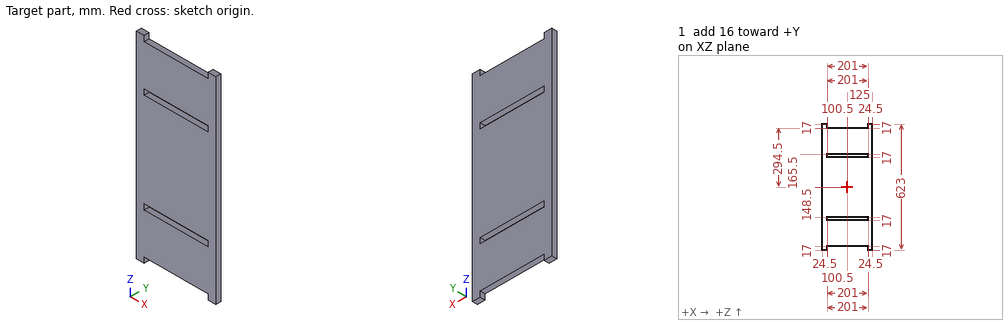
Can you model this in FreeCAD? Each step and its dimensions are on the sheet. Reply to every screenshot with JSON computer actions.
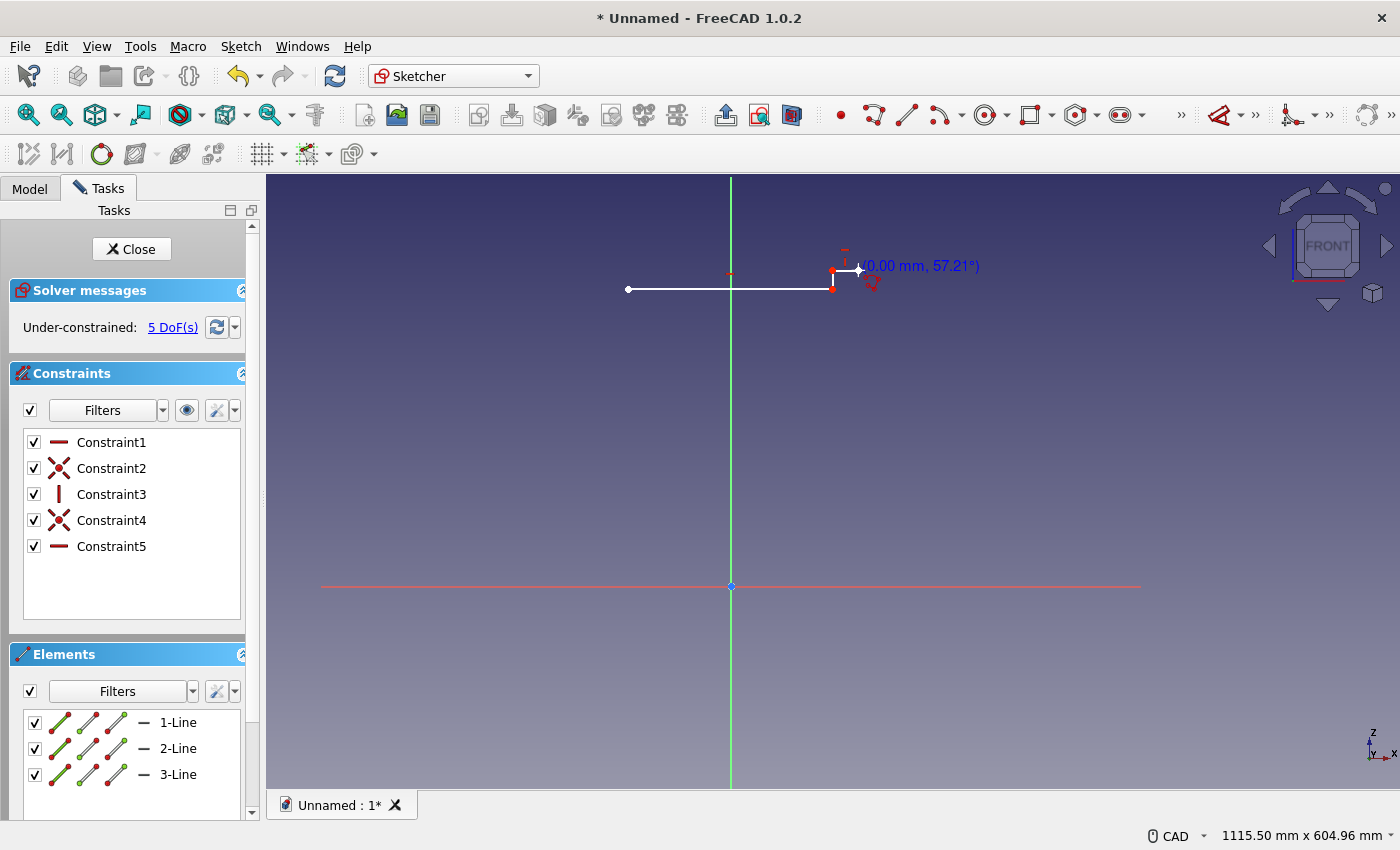
{"action": "scroll", "coordinate": [832, 267], "scroll_direction": "down", "scroll_amount": 2}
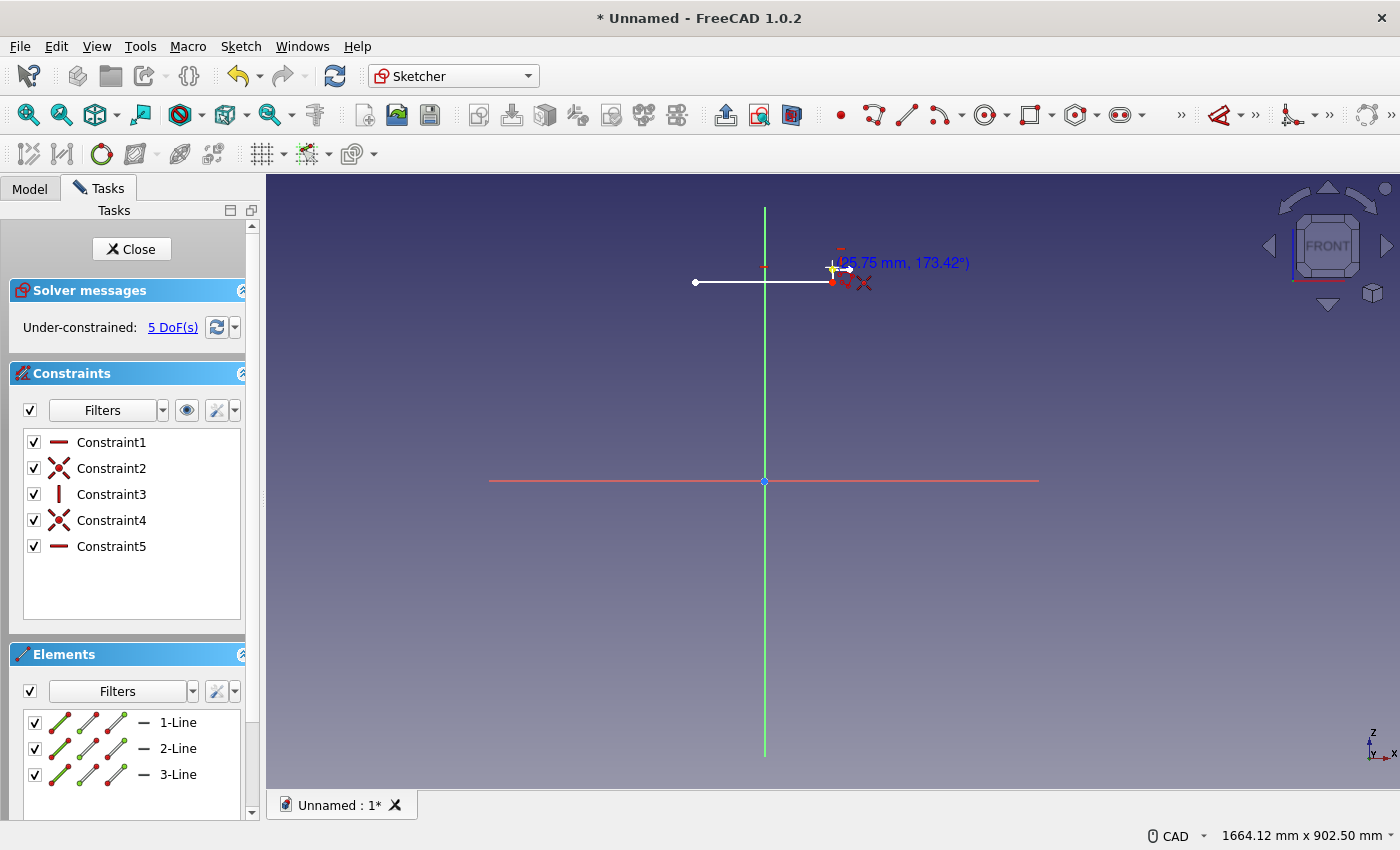
{"action": "left_click", "coordinate": [850, 694]}
{"action": "left_click", "coordinate": [833, 694]}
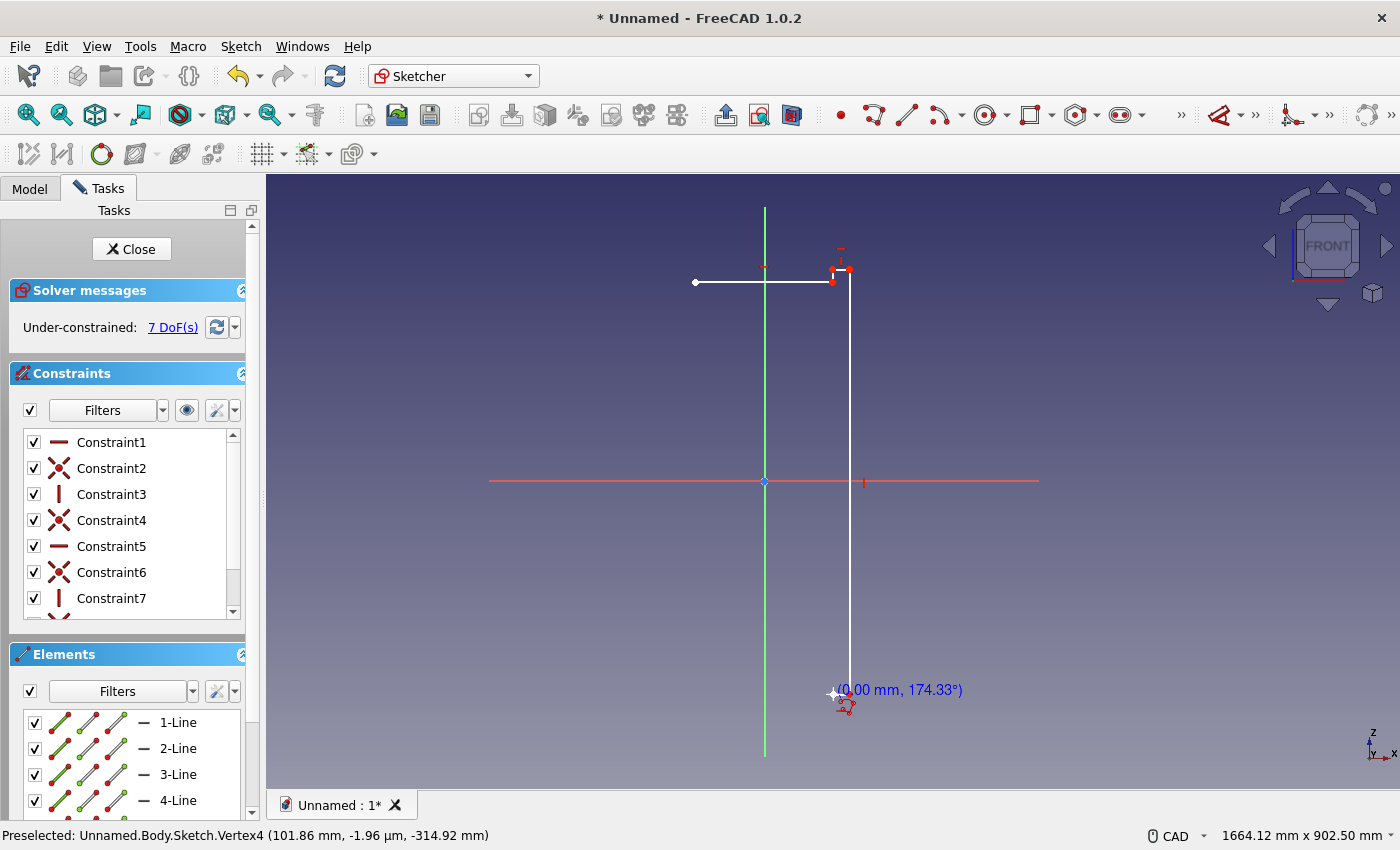
{"action": "scroll", "coordinate": [833, 682], "scroll_direction": "up", "scroll_amount": 2}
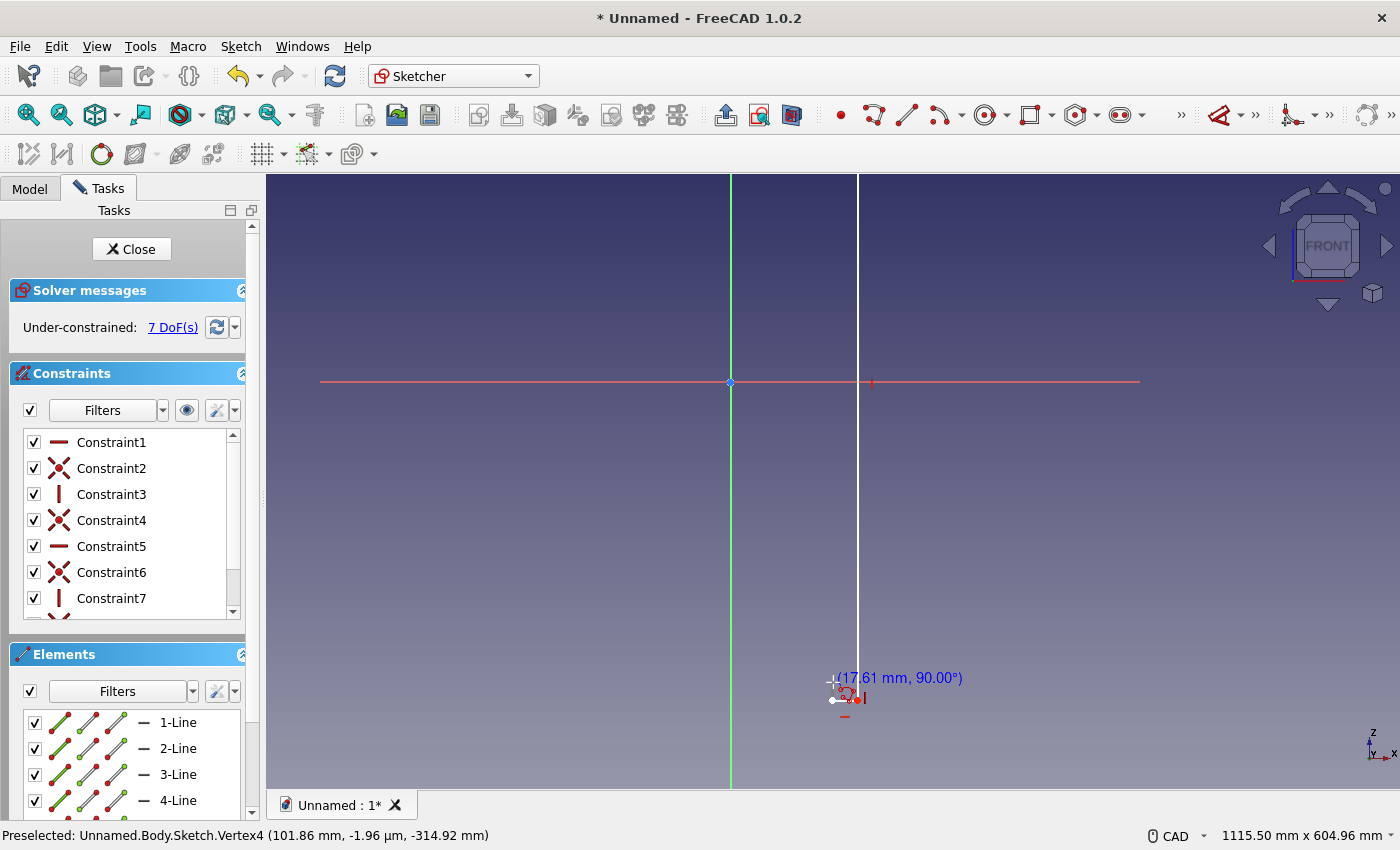
{"action": "left_click", "coordinate": [833, 682]}
{"action": "left_click", "coordinate": [629, 682]}
{"action": "left_click", "coordinate": [629, 699]}
{"action": "left_click", "coordinate": [604, 699]}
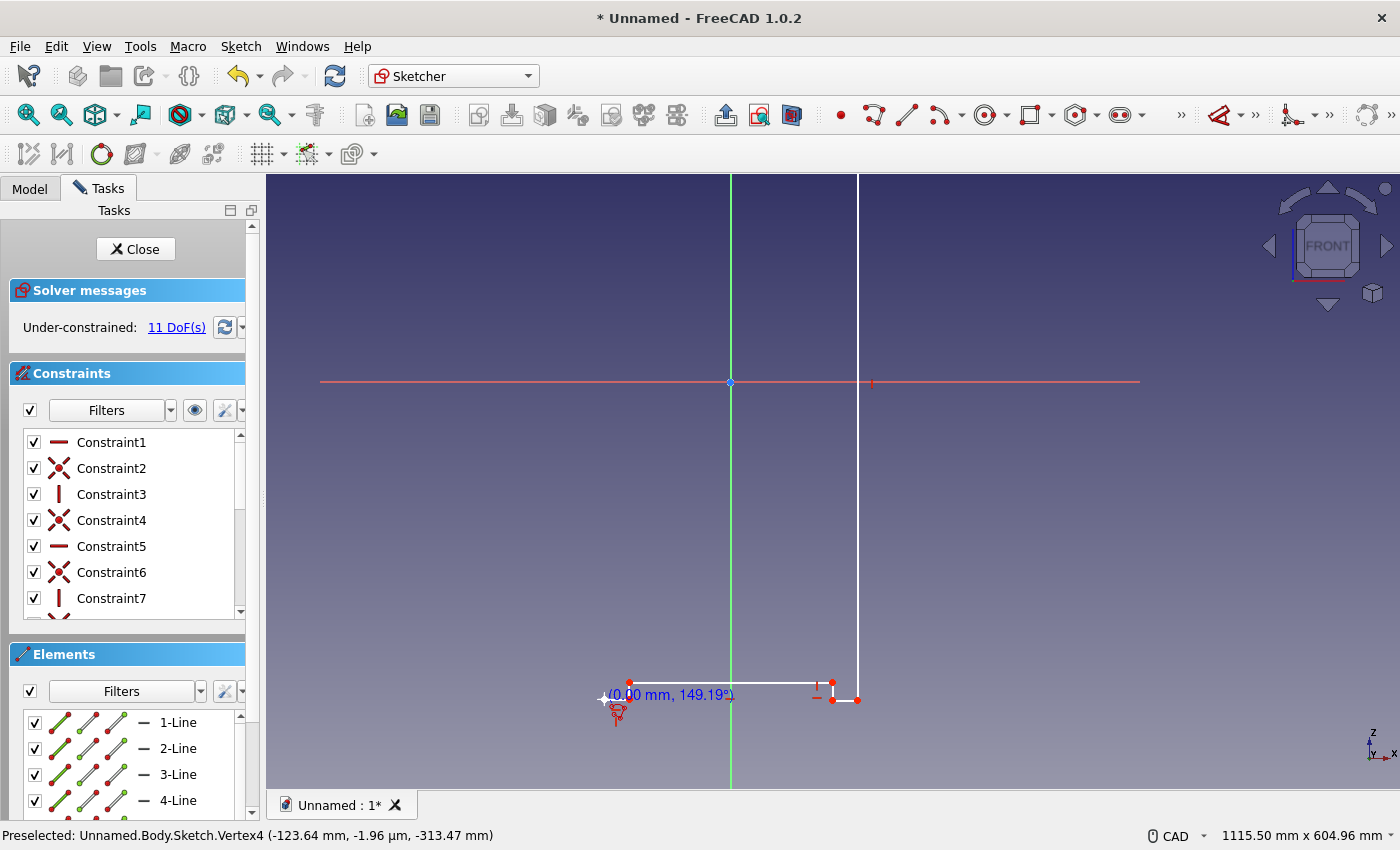
{"action": "scroll", "coordinate": [833, 683], "scroll_direction": "down", "scroll_amount": 2}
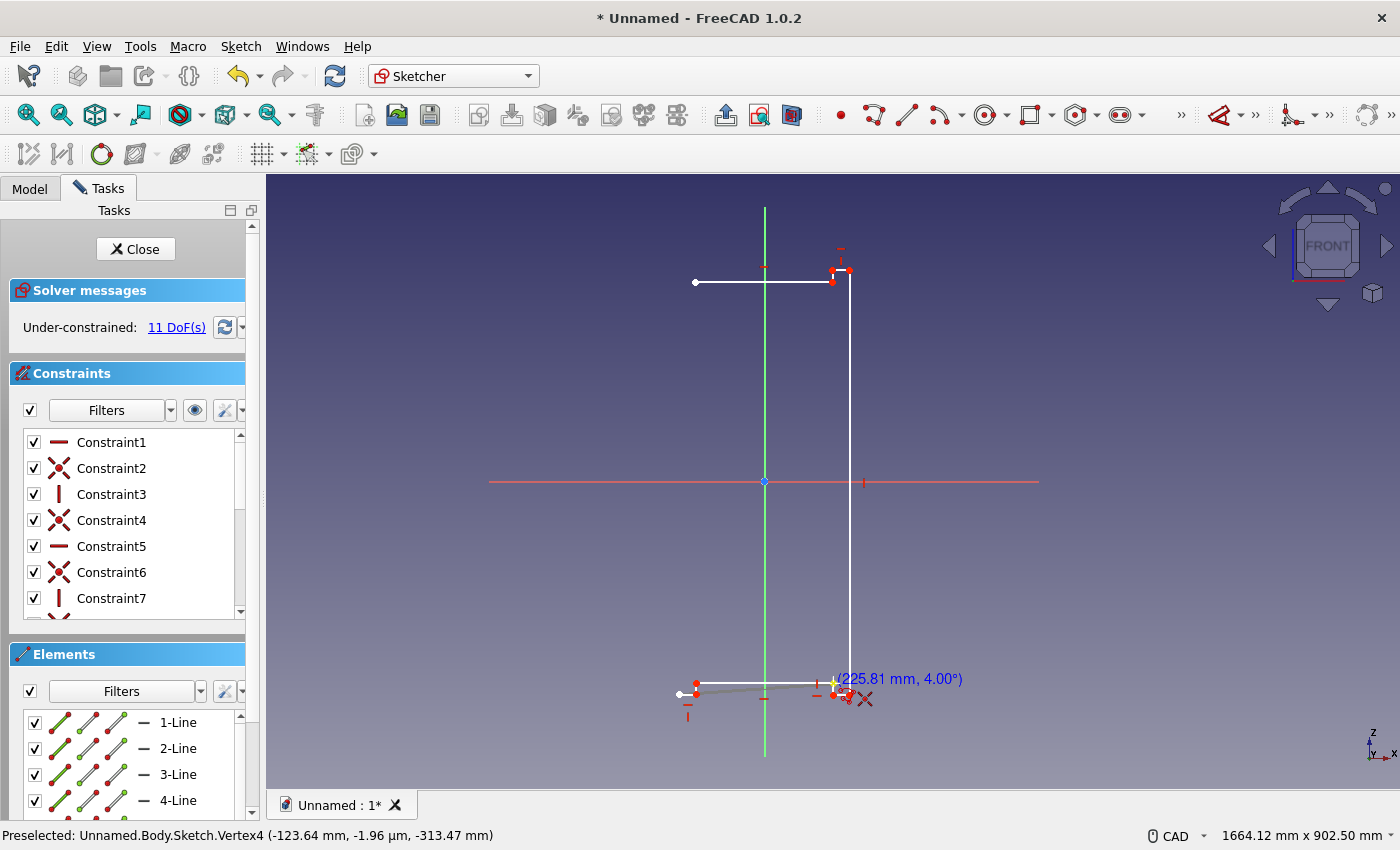
{"action": "left_click", "coordinate": [680, 269]}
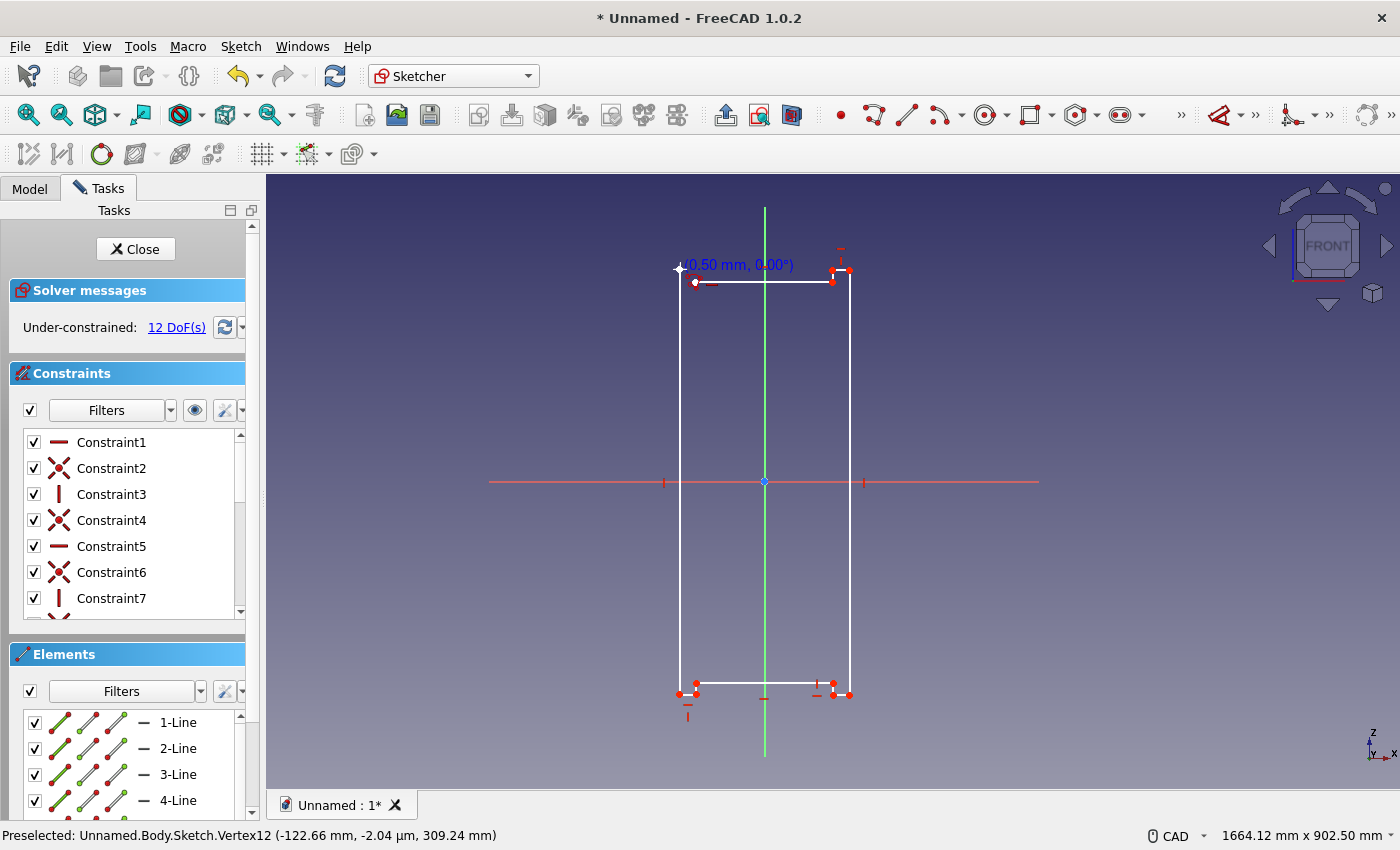
{"action": "scroll", "coordinate": [696, 269], "scroll_direction": "up", "scroll_amount": 2}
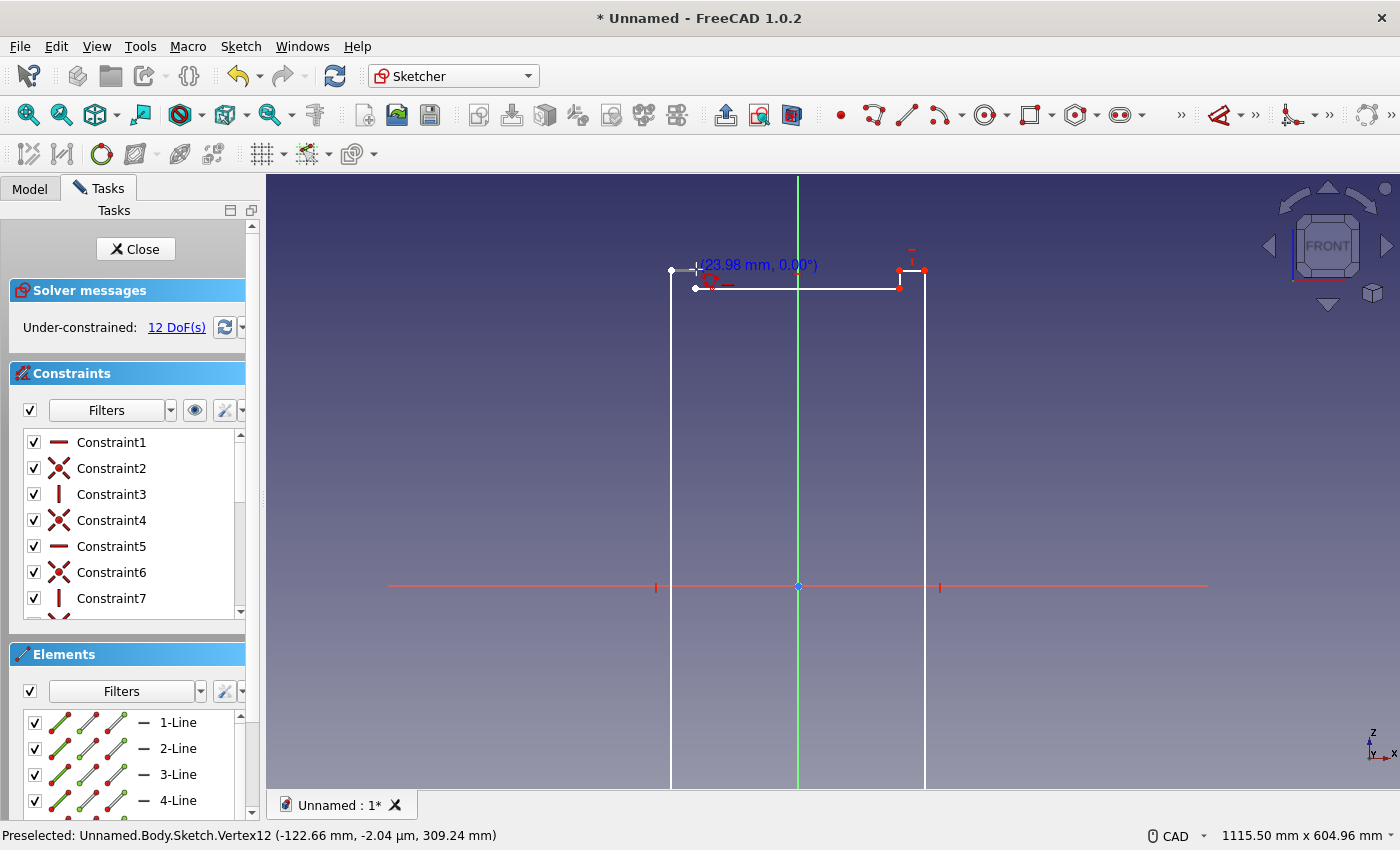
{"action": "left_click", "coordinate": [696, 269]}
{"action": "left_click", "coordinate": [695, 289]}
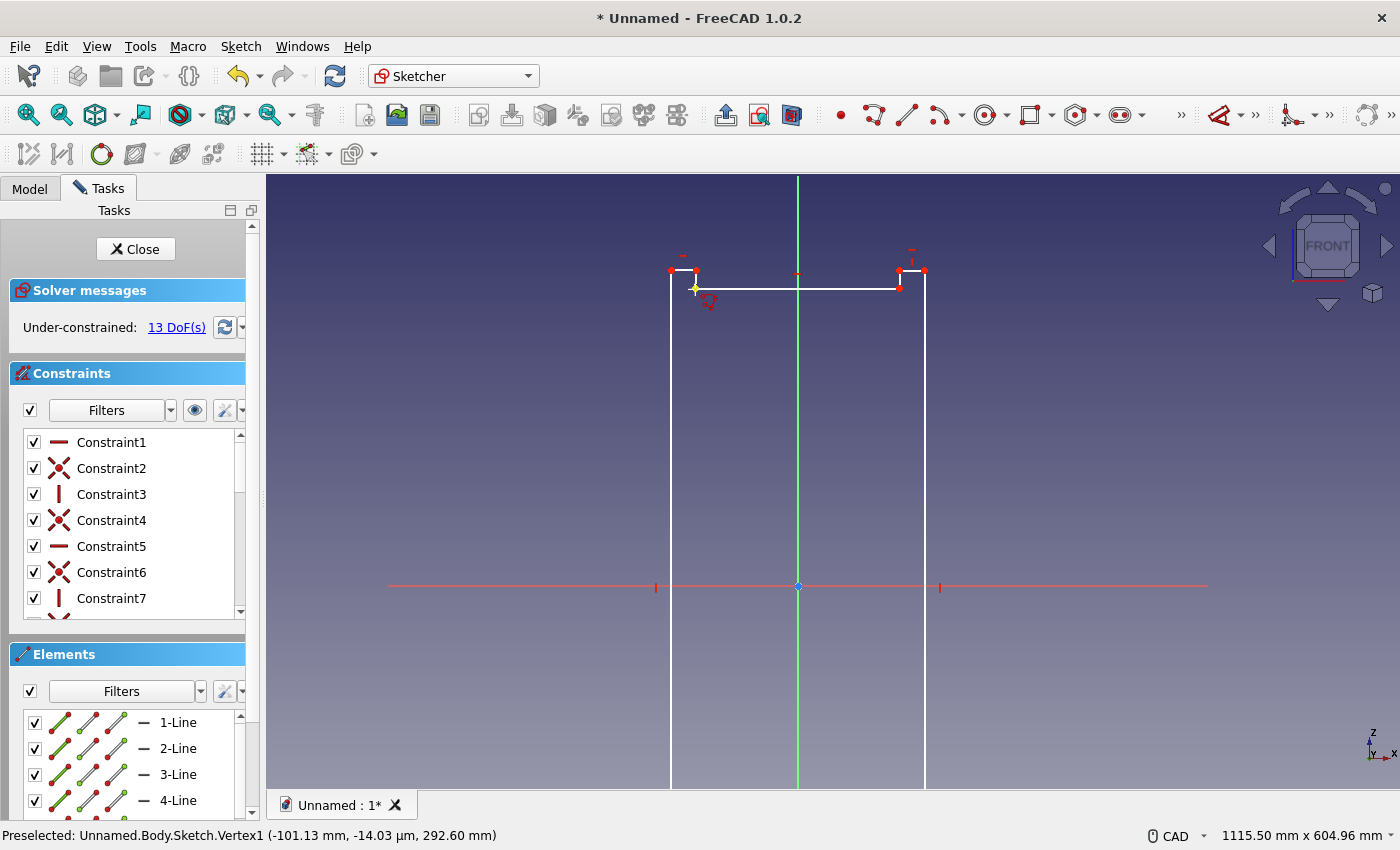
{"action": "key", "text": "g r"}